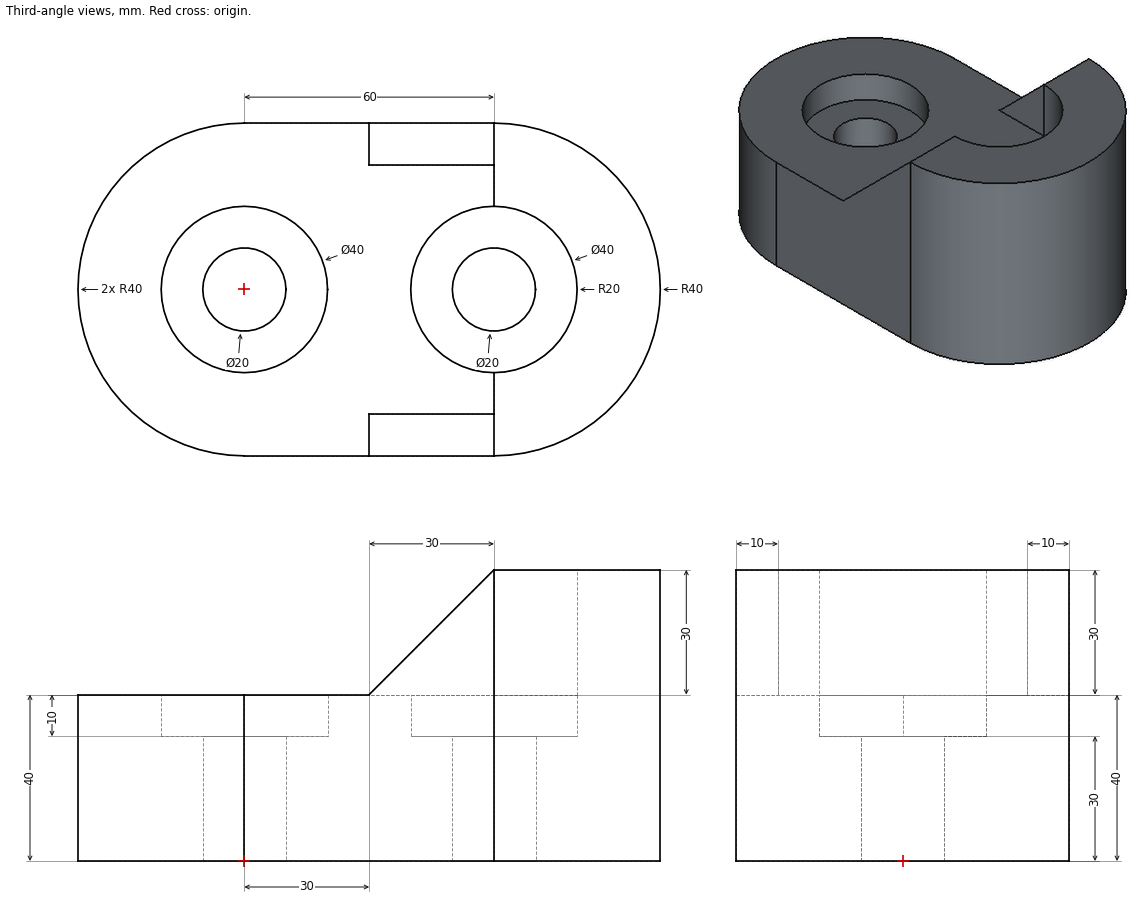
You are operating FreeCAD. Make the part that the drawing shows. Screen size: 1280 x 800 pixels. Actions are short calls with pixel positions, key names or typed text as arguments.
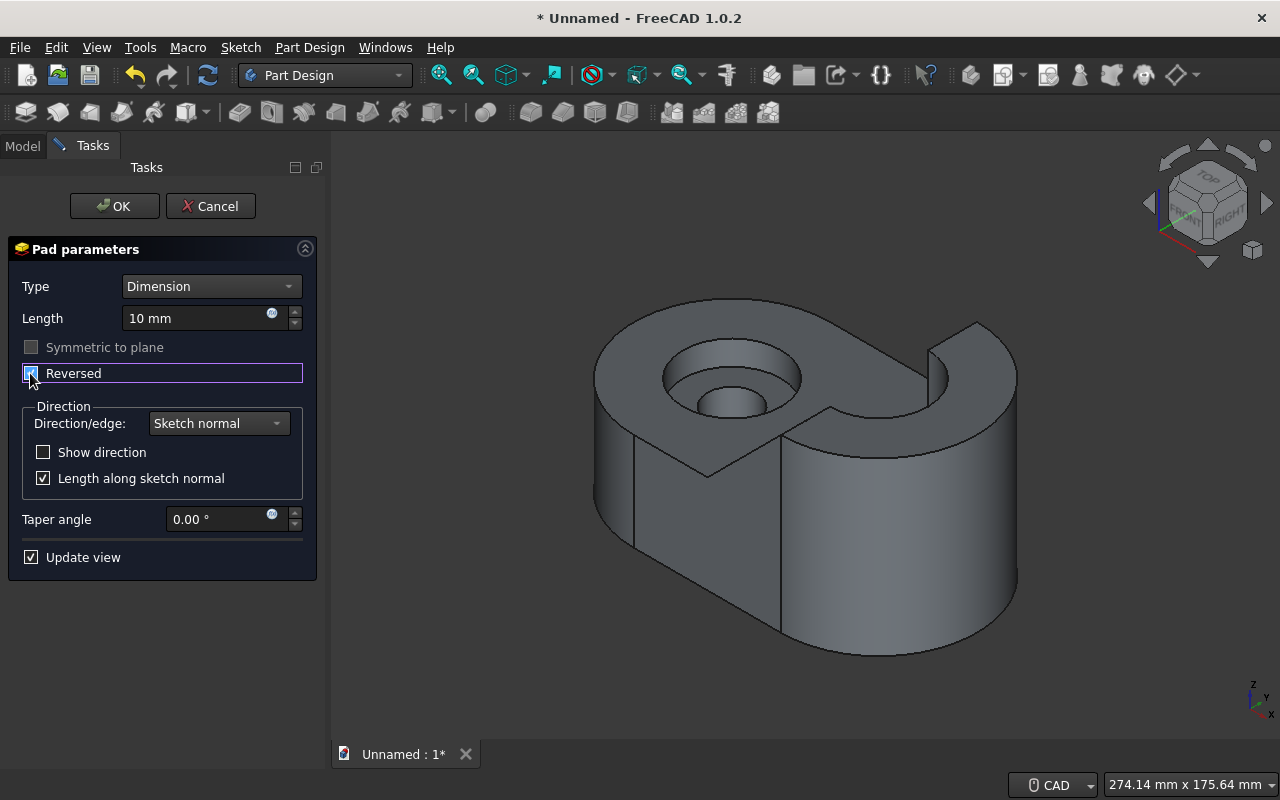
click(115, 206)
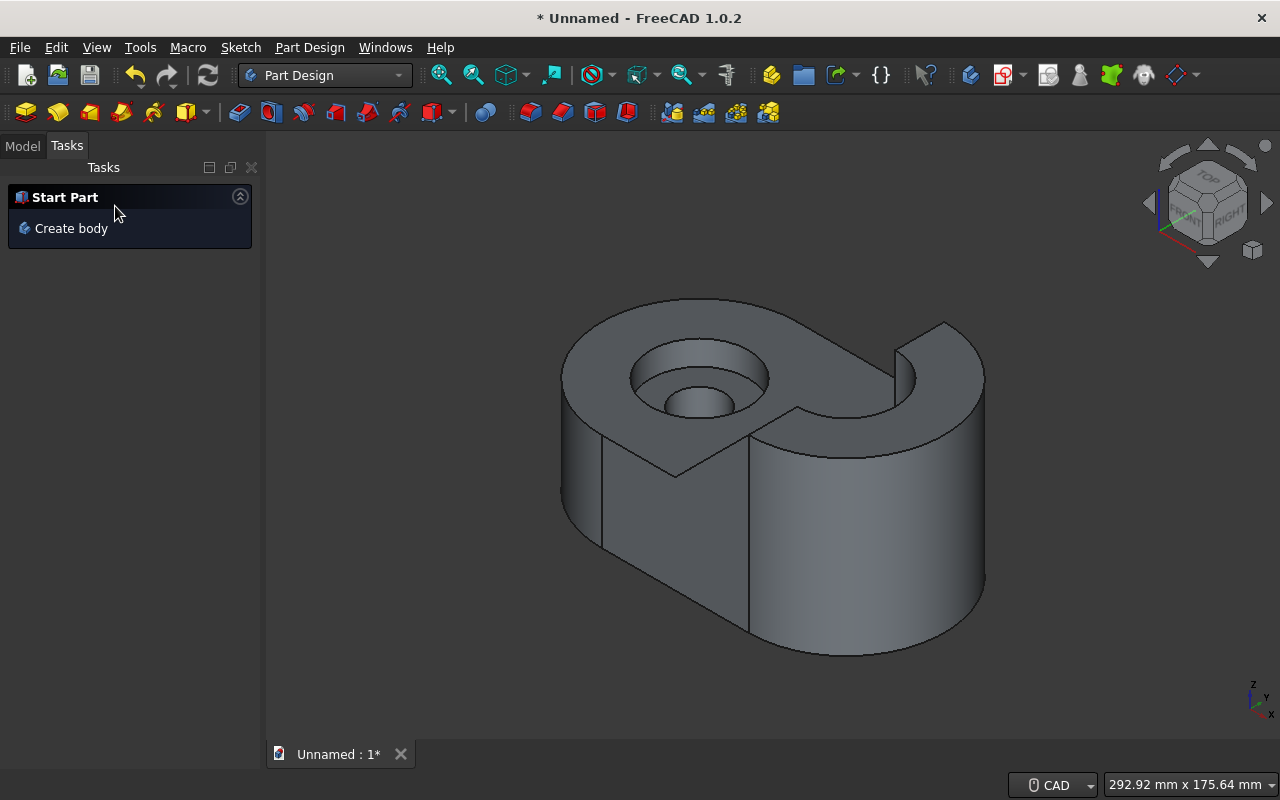
key(4)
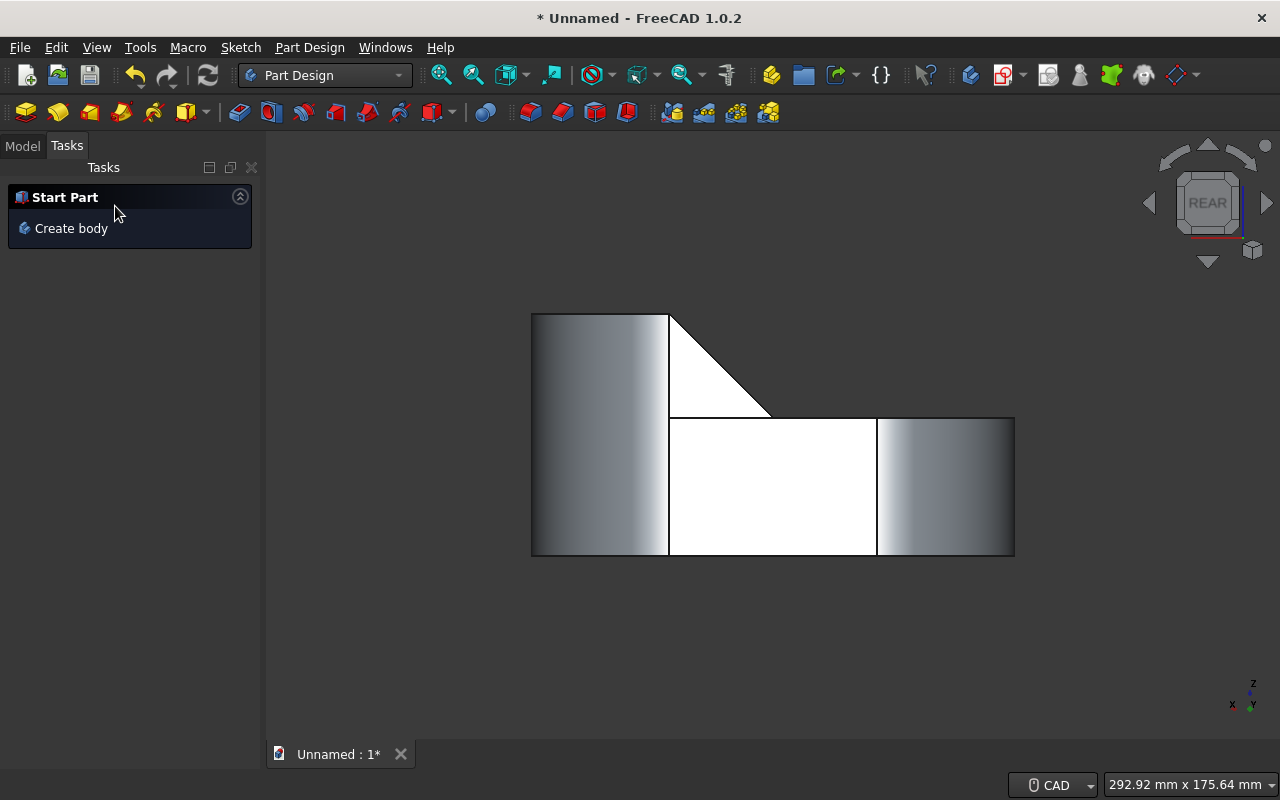
click(743, 486)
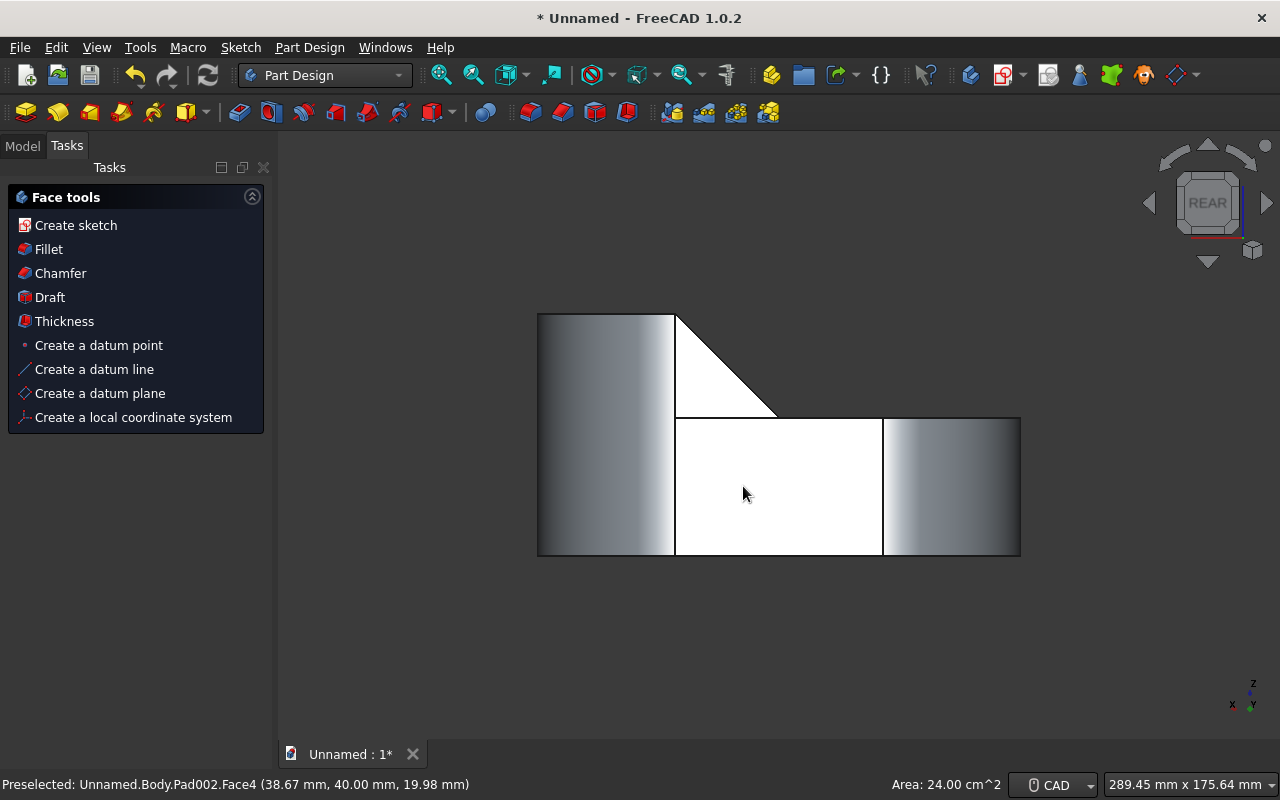
click(1004, 76)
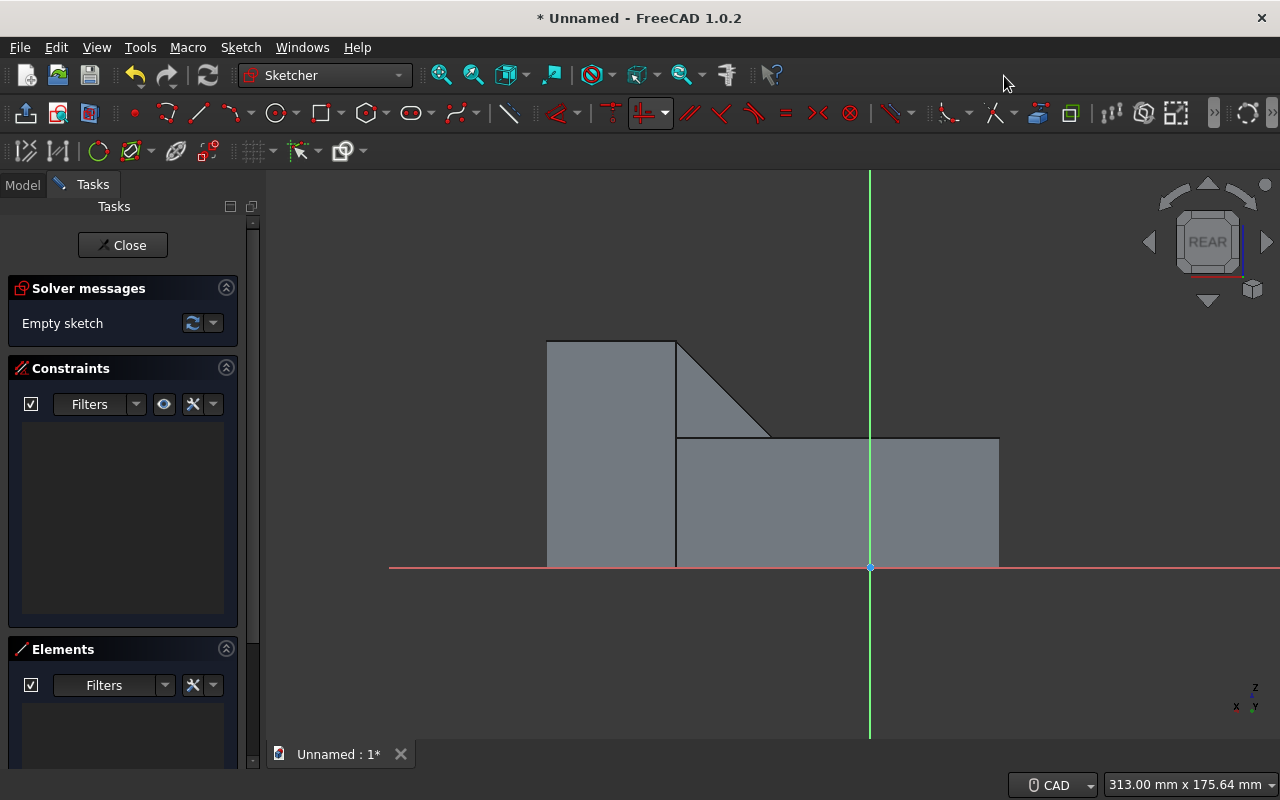
scroll(912, 454, up, 2)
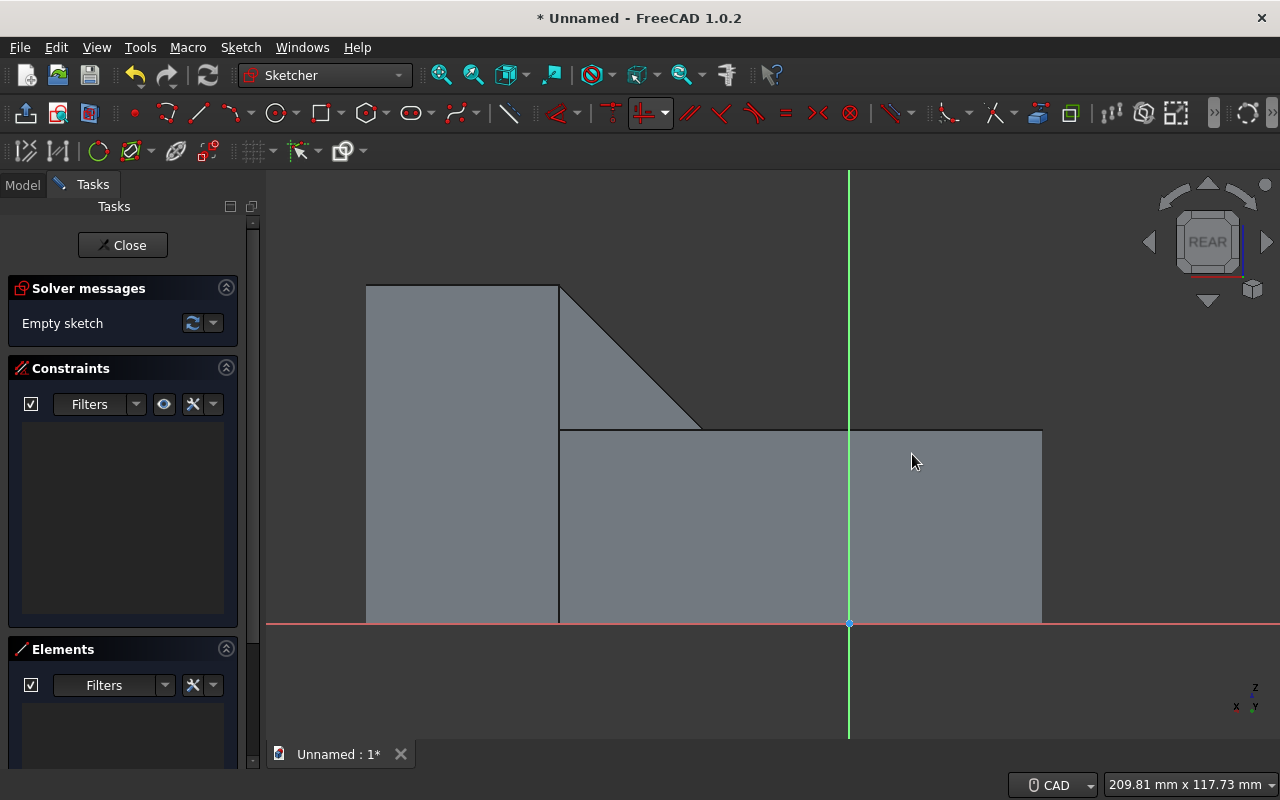
click(168, 114)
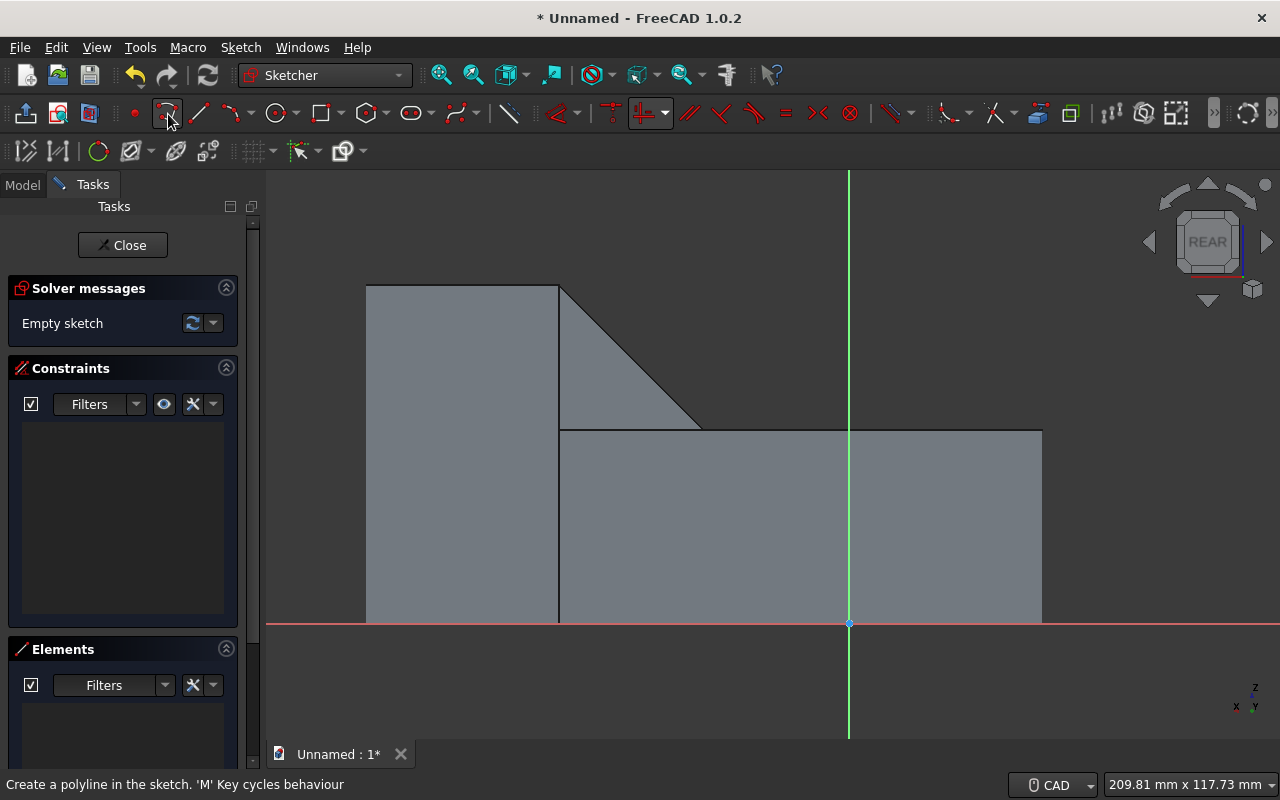
click(704, 430)
click(559, 285)
click(559, 430)
click(704, 431)
key(Escape)
key(Escape)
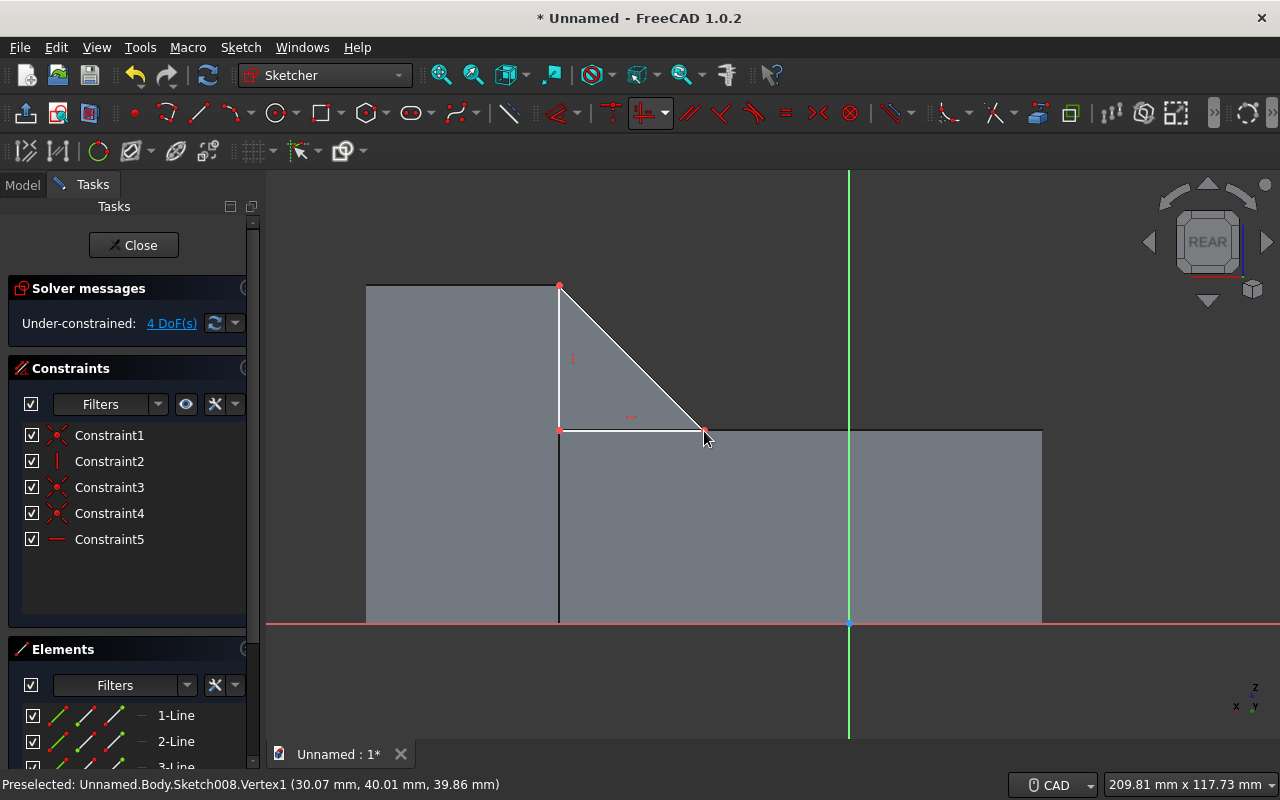
click(556, 114)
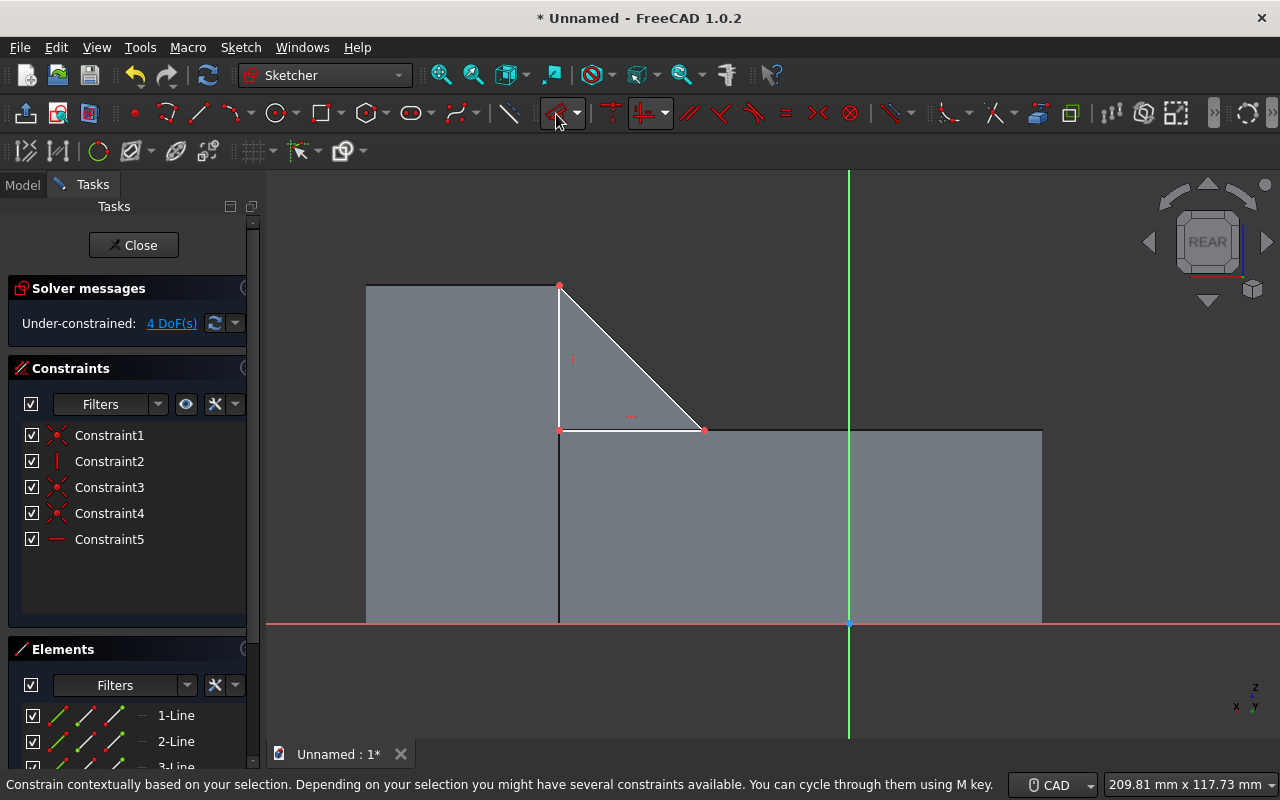
click(559, 329)
click(525, 359)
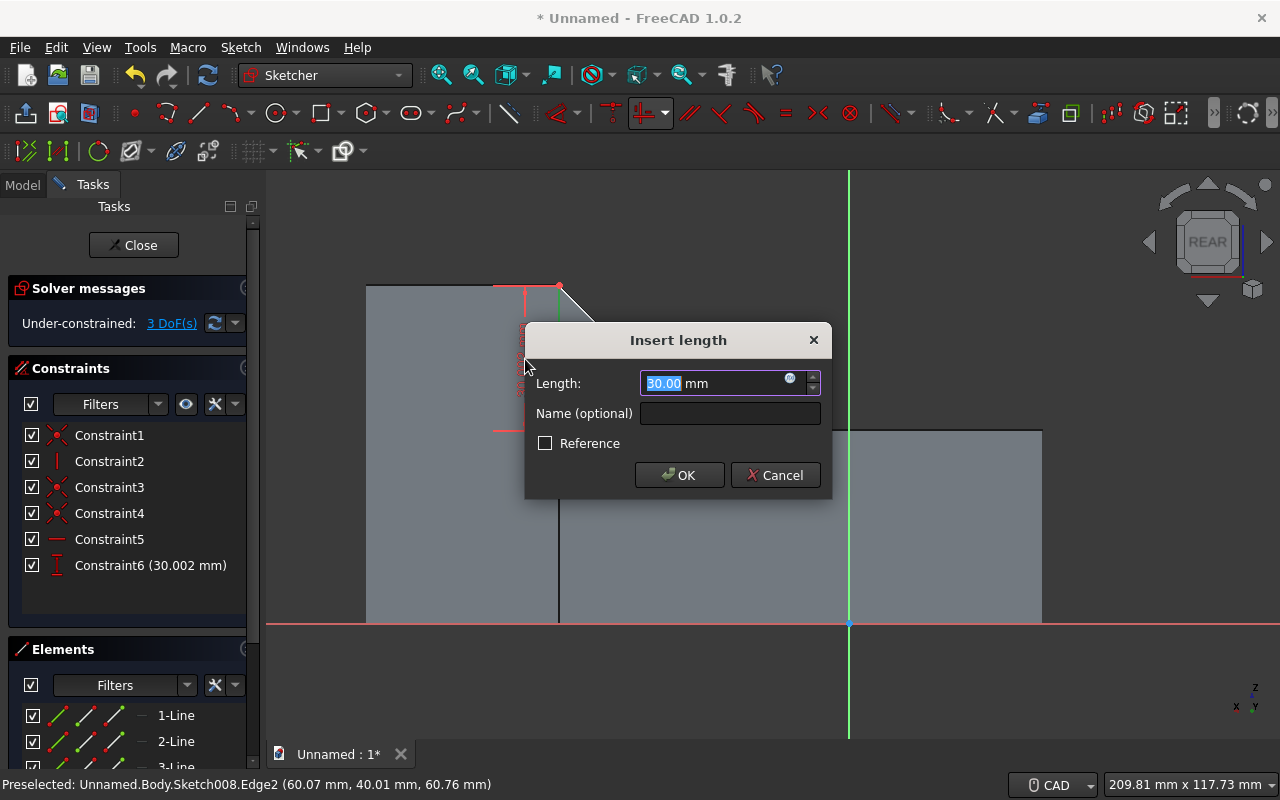
text(30)
key(Return)